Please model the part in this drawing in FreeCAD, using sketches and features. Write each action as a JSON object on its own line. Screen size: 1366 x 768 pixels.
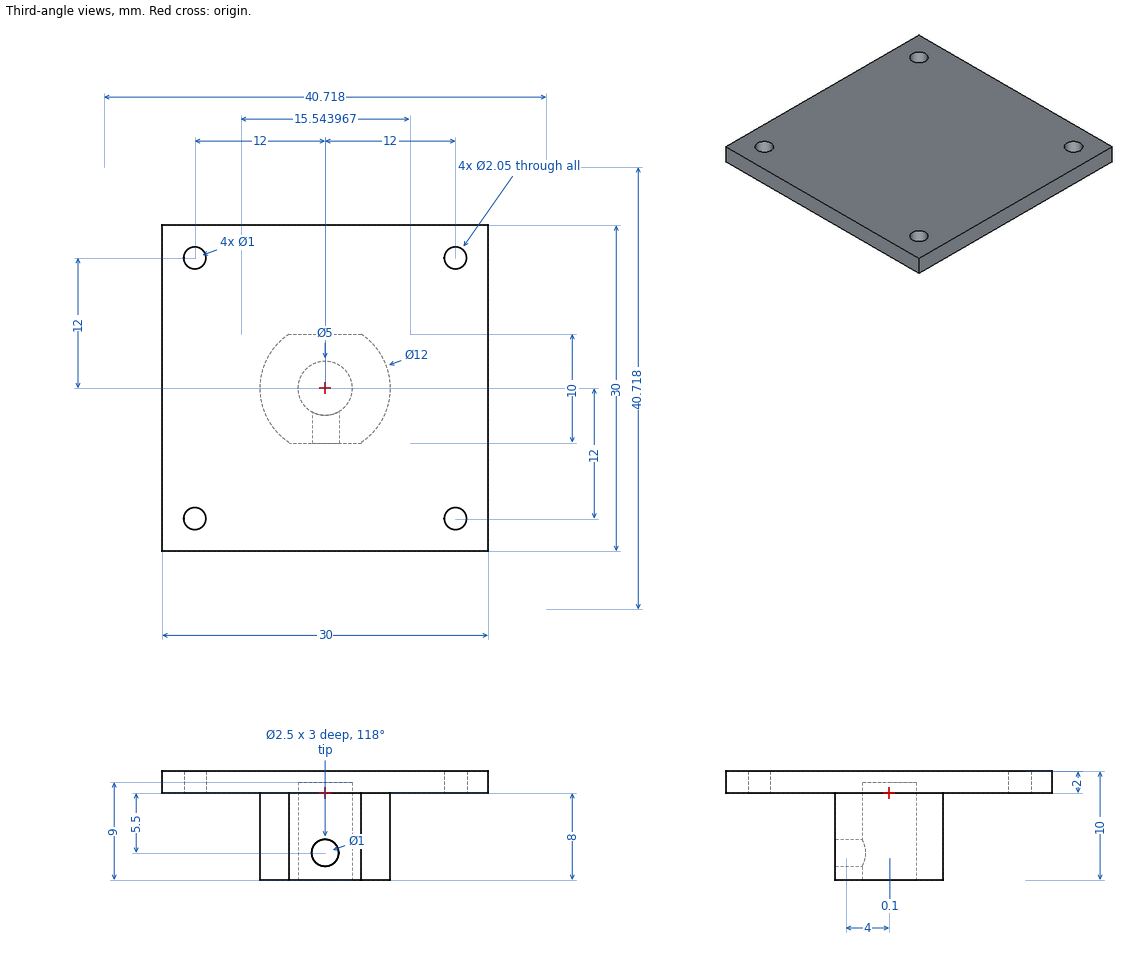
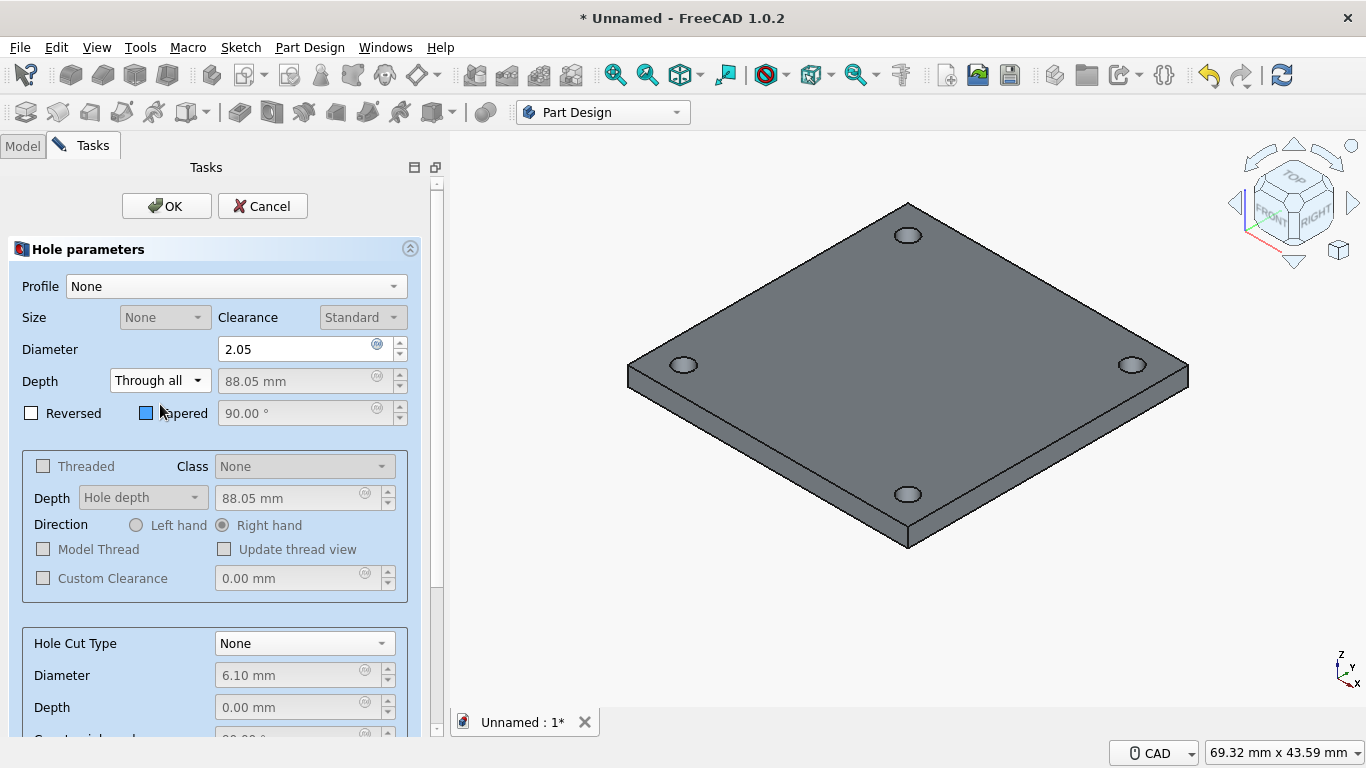
{"action": "left_click", "coordinate": [167, 206]}